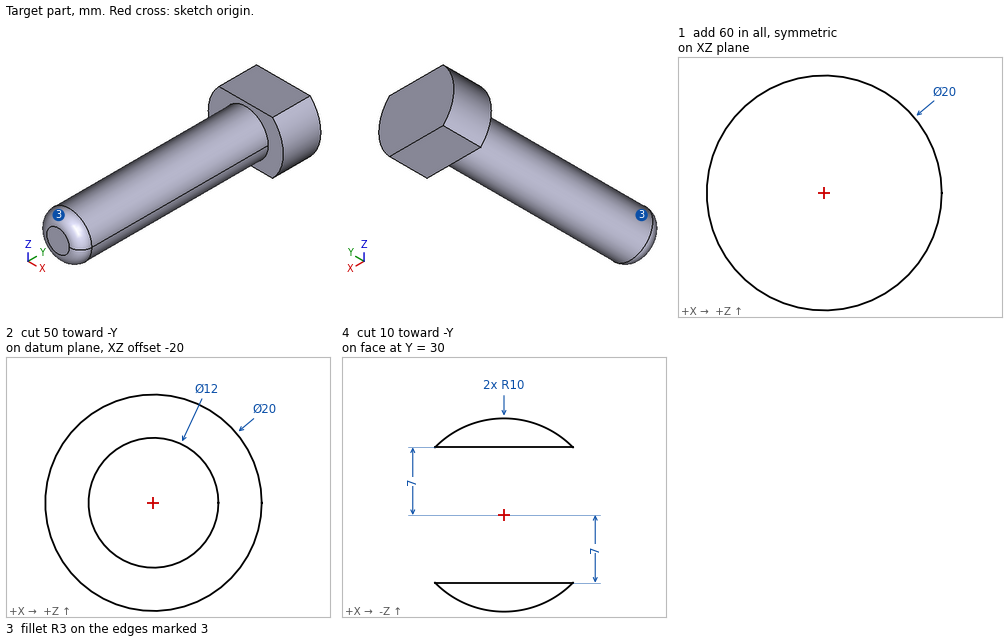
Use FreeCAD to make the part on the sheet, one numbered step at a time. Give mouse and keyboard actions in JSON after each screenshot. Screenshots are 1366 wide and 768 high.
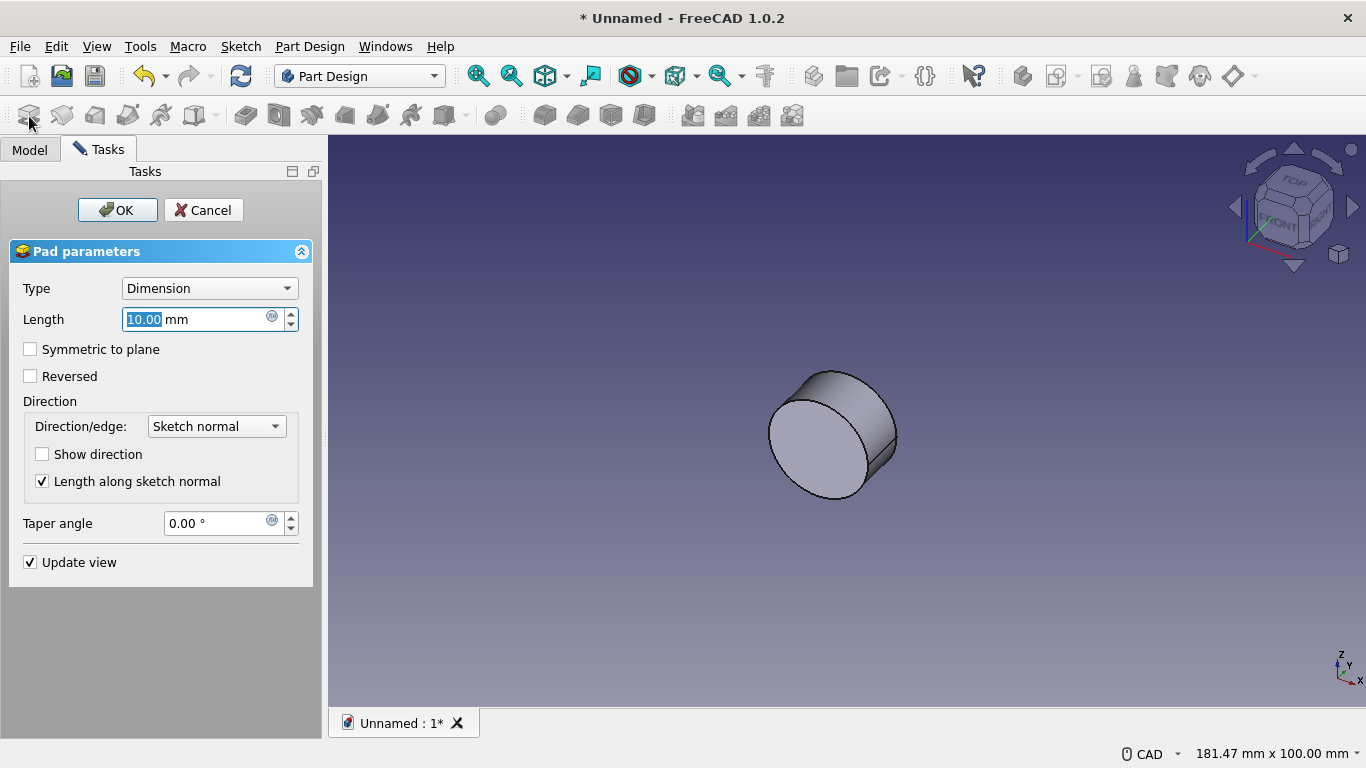
{"action": "type", "text": "60"}
{"action": "key", "text": "Tab"}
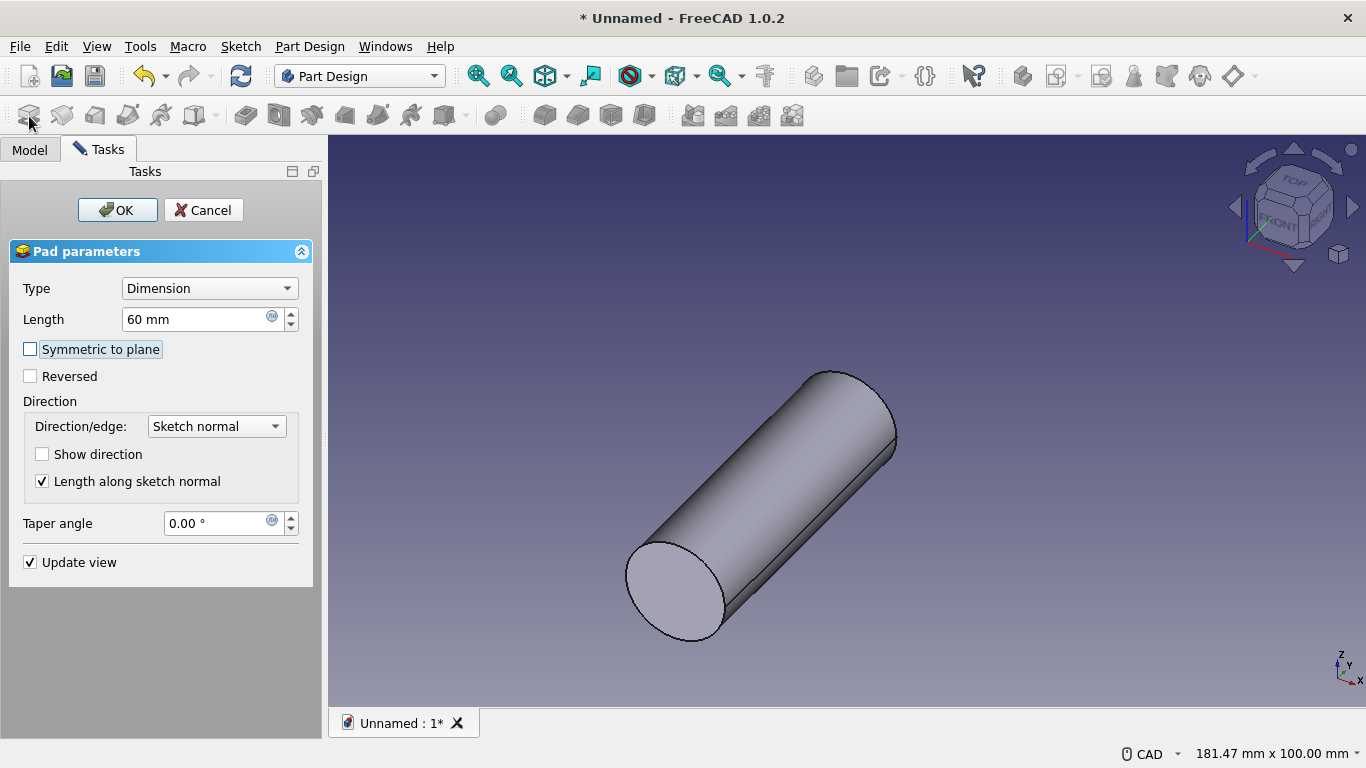
{"action": "left_click", "coordinate": [31, 349]}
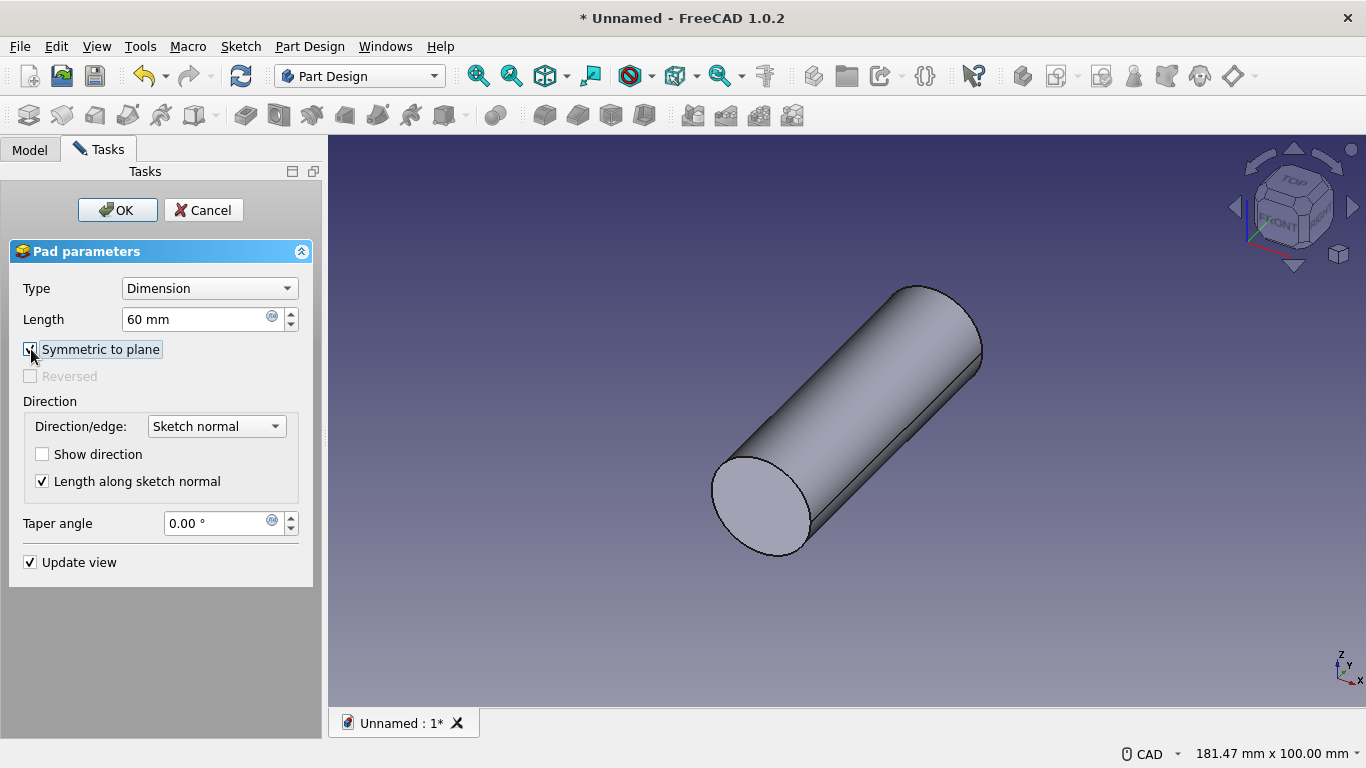
{"action": "left_click", "coordinate": [118, 210]}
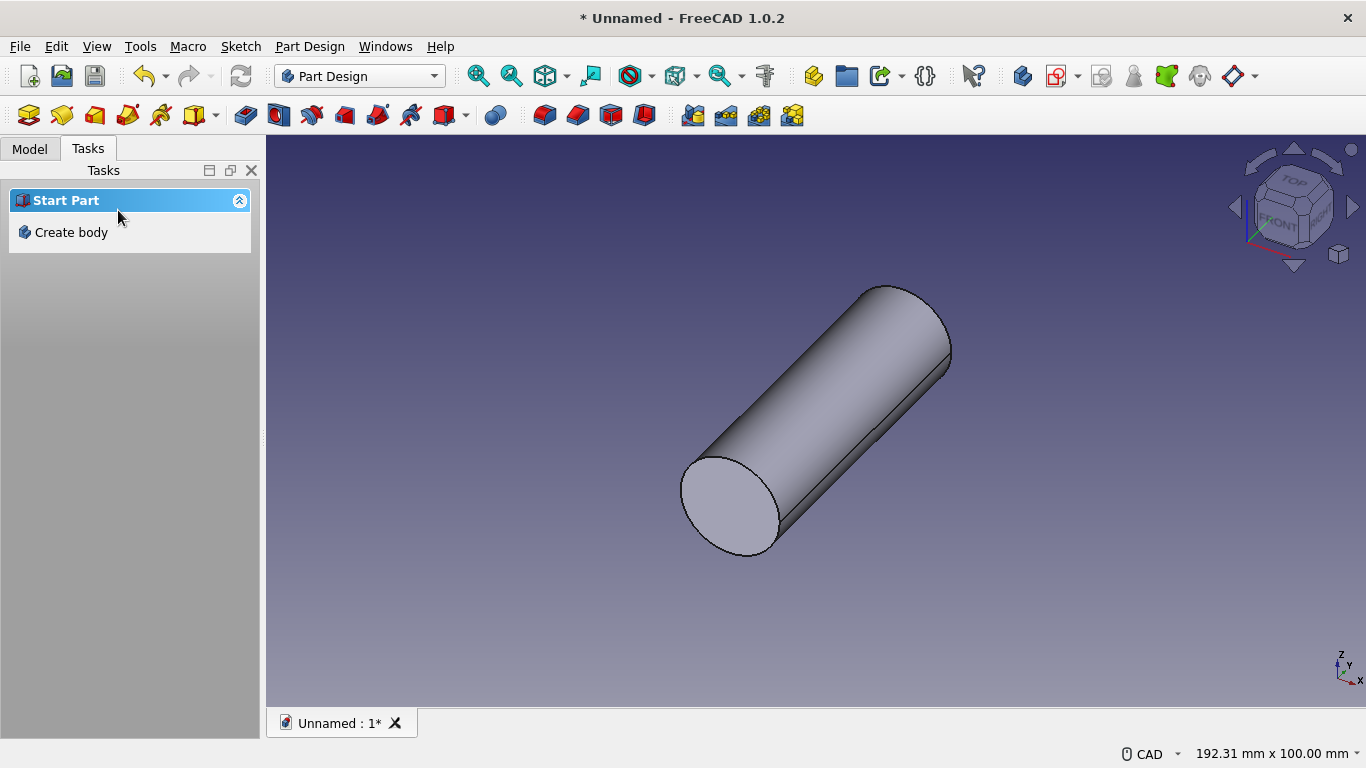
{"action": "left_click", "coordinate": [30, 148]}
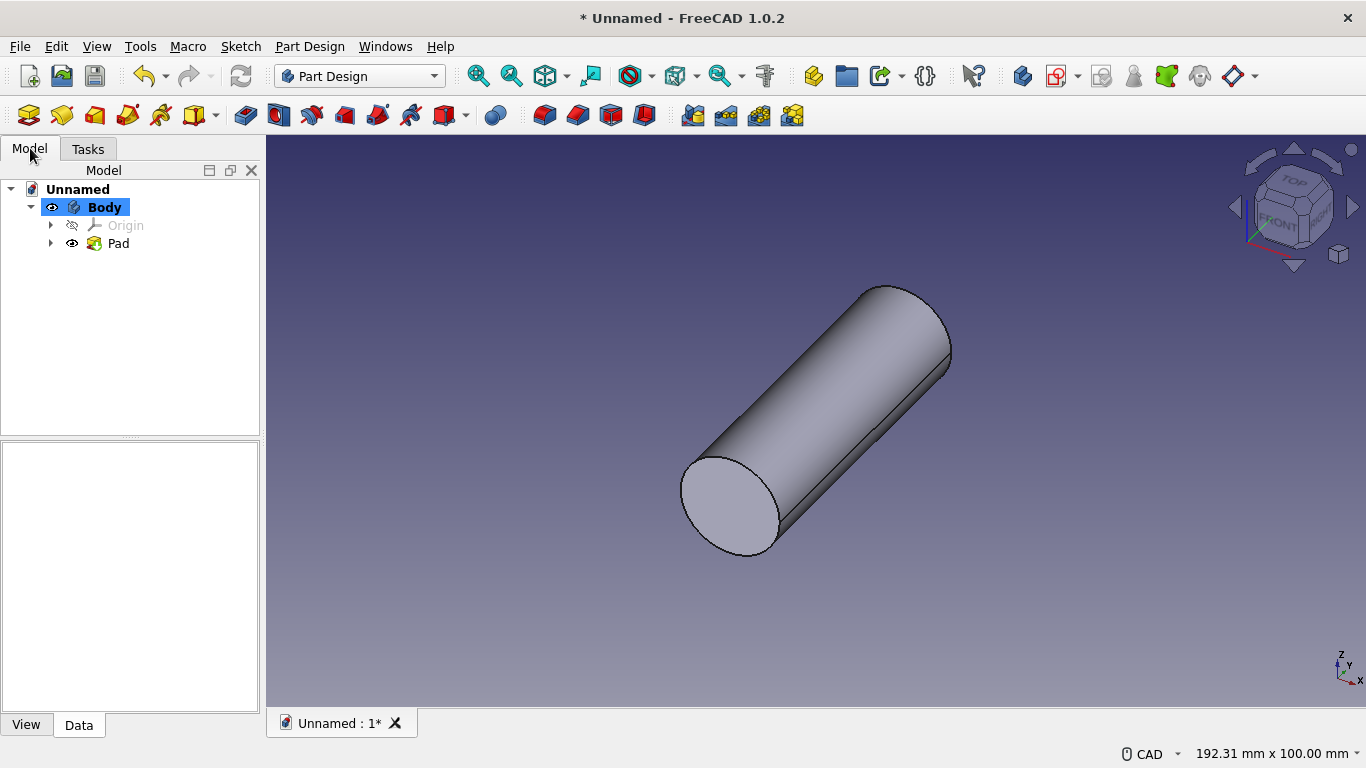
{"action": "left_click", "coordinate": [51, 225]}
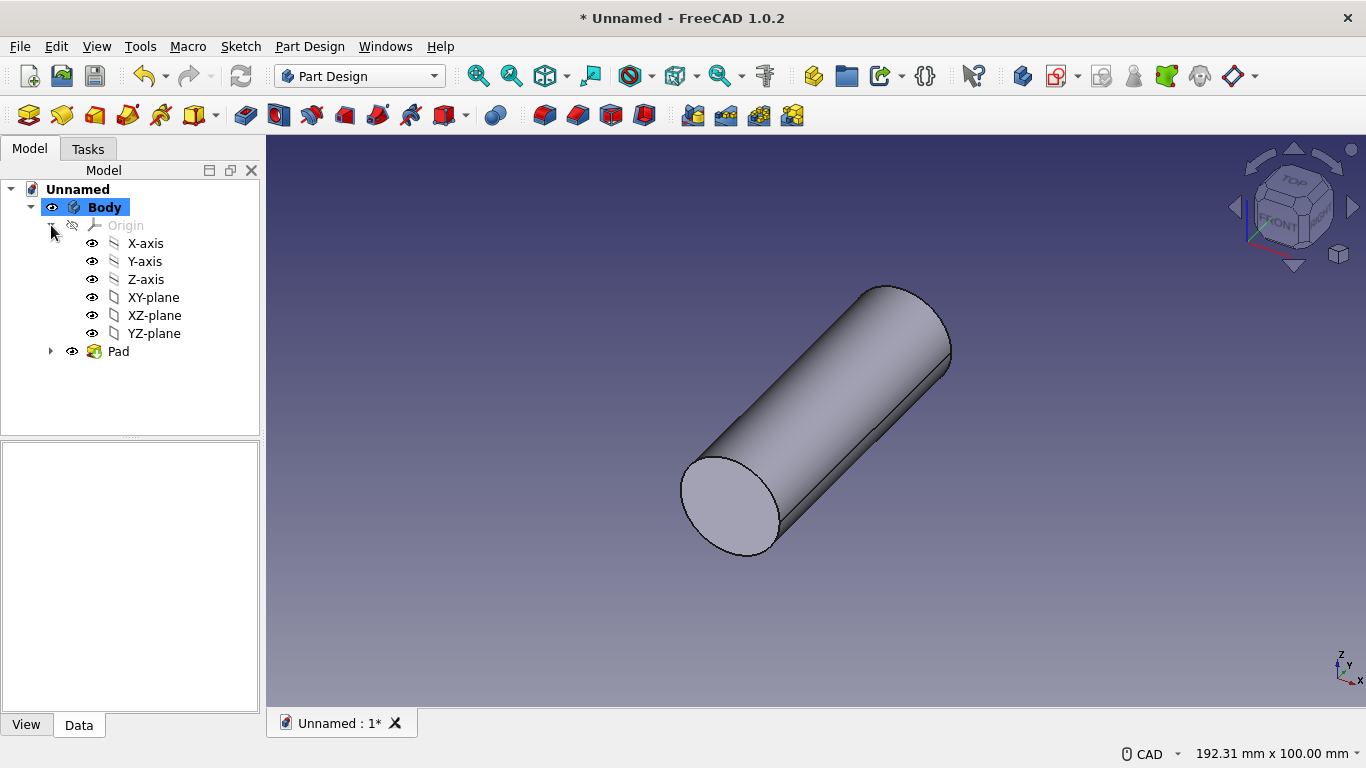
{"action": "left_click", "coordinate": [137, 315]}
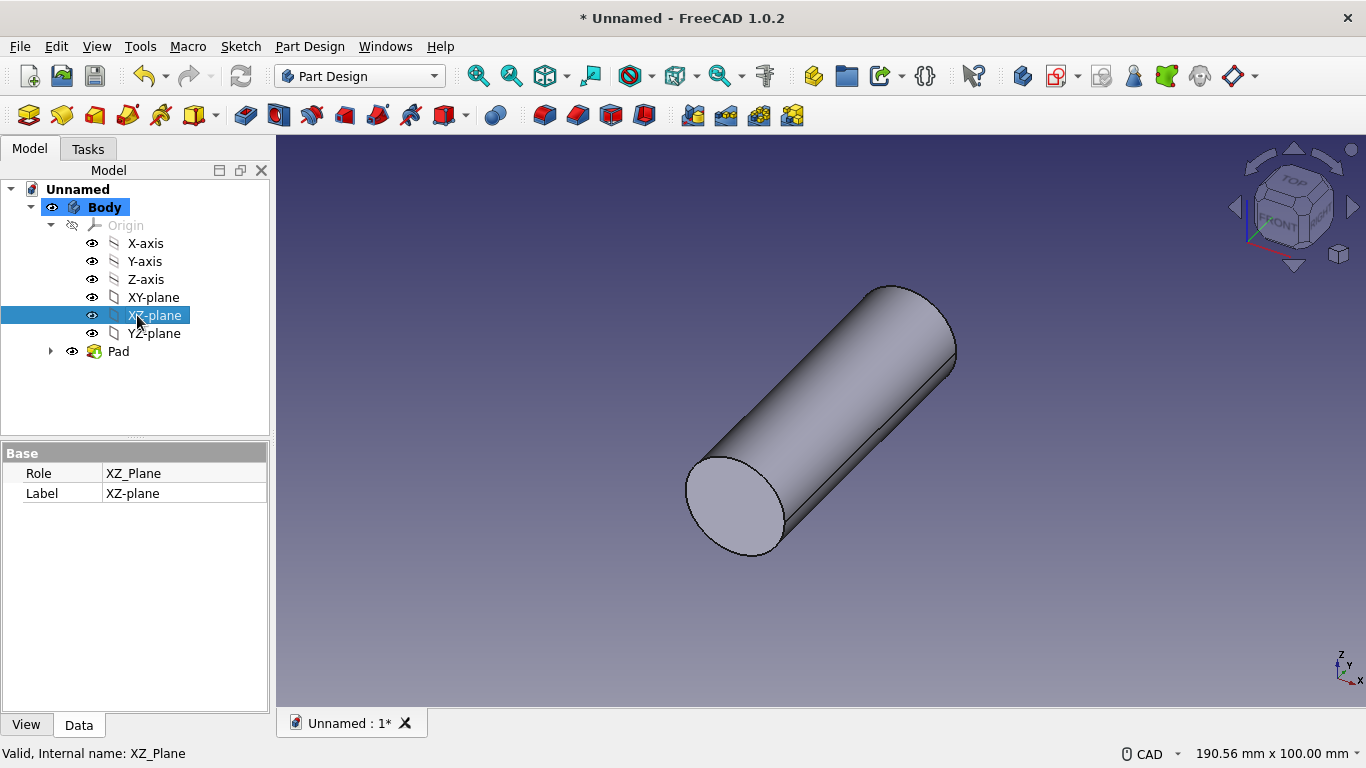
{"action": "left_click", "coordinate": [1232, 76]}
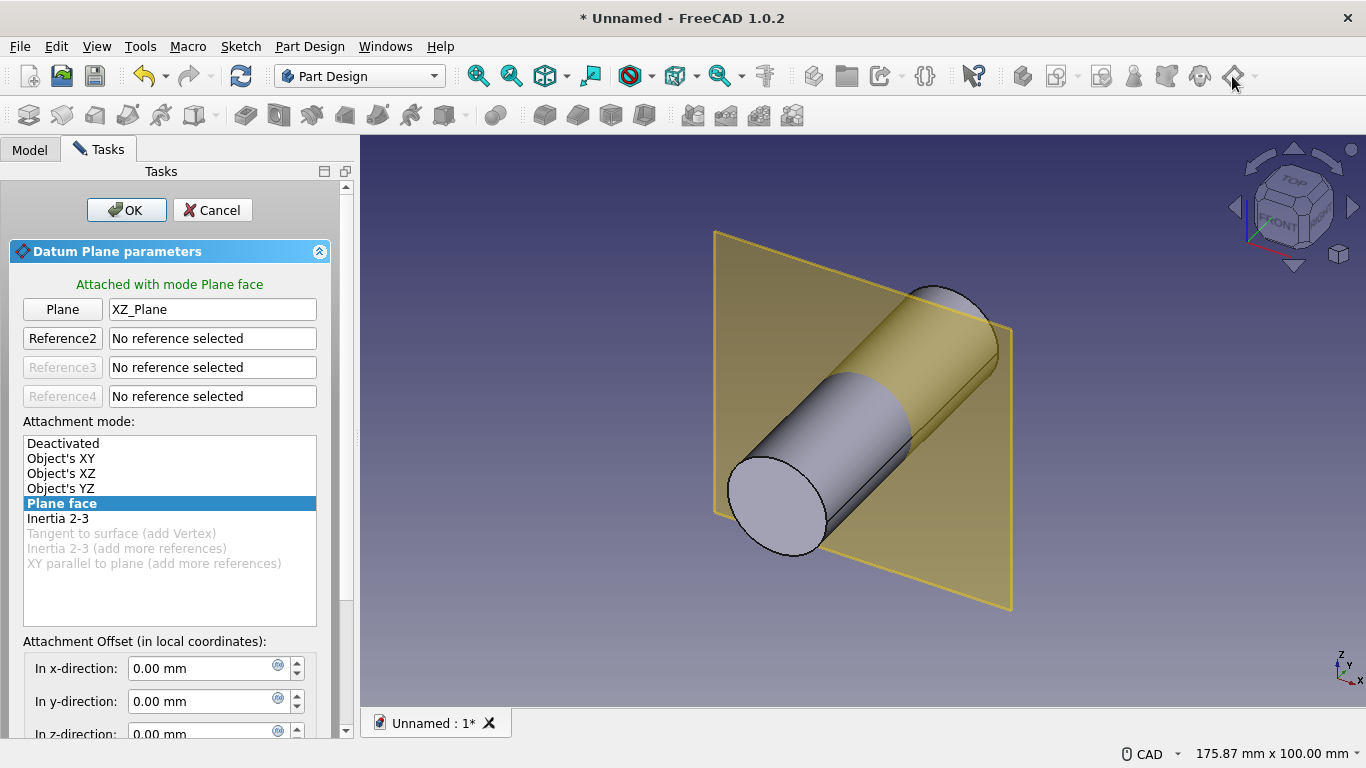
{"action": "scroll", "coordinate": [346, 460], "scroll_direction": "down", "scroll_amount": 2}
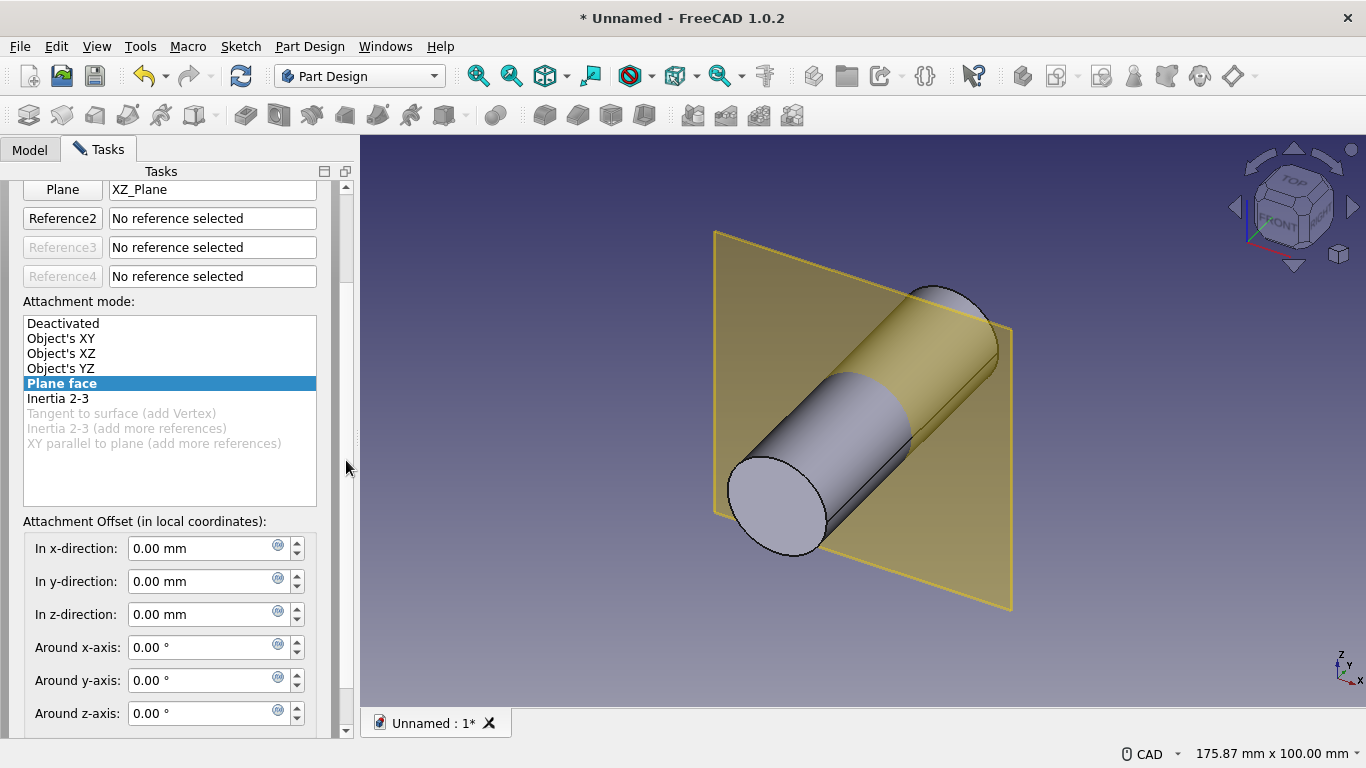
{"action": "triple_click", "coordinate": [210, 614]}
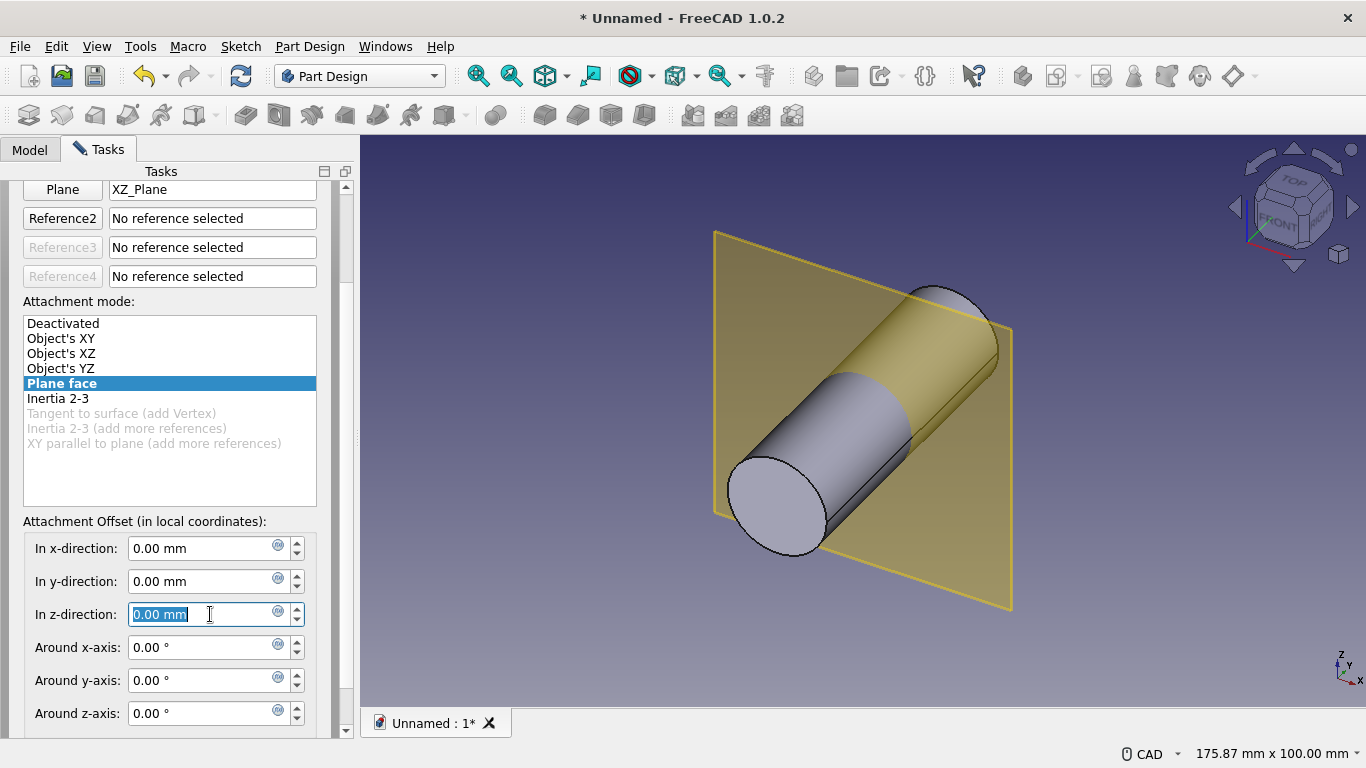
{"action": "type", "text": "-20"}
{"action": "key", "text": "Tab"}